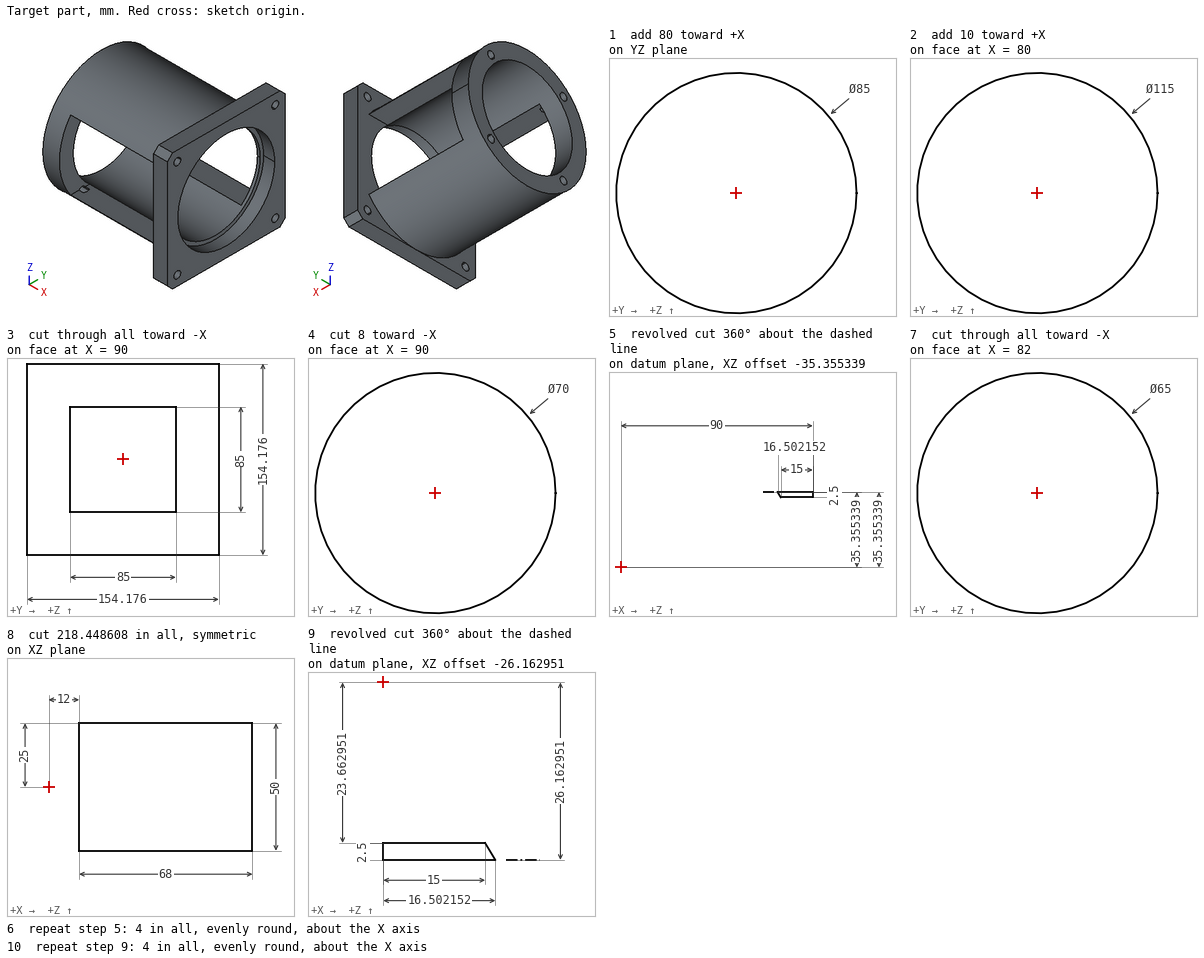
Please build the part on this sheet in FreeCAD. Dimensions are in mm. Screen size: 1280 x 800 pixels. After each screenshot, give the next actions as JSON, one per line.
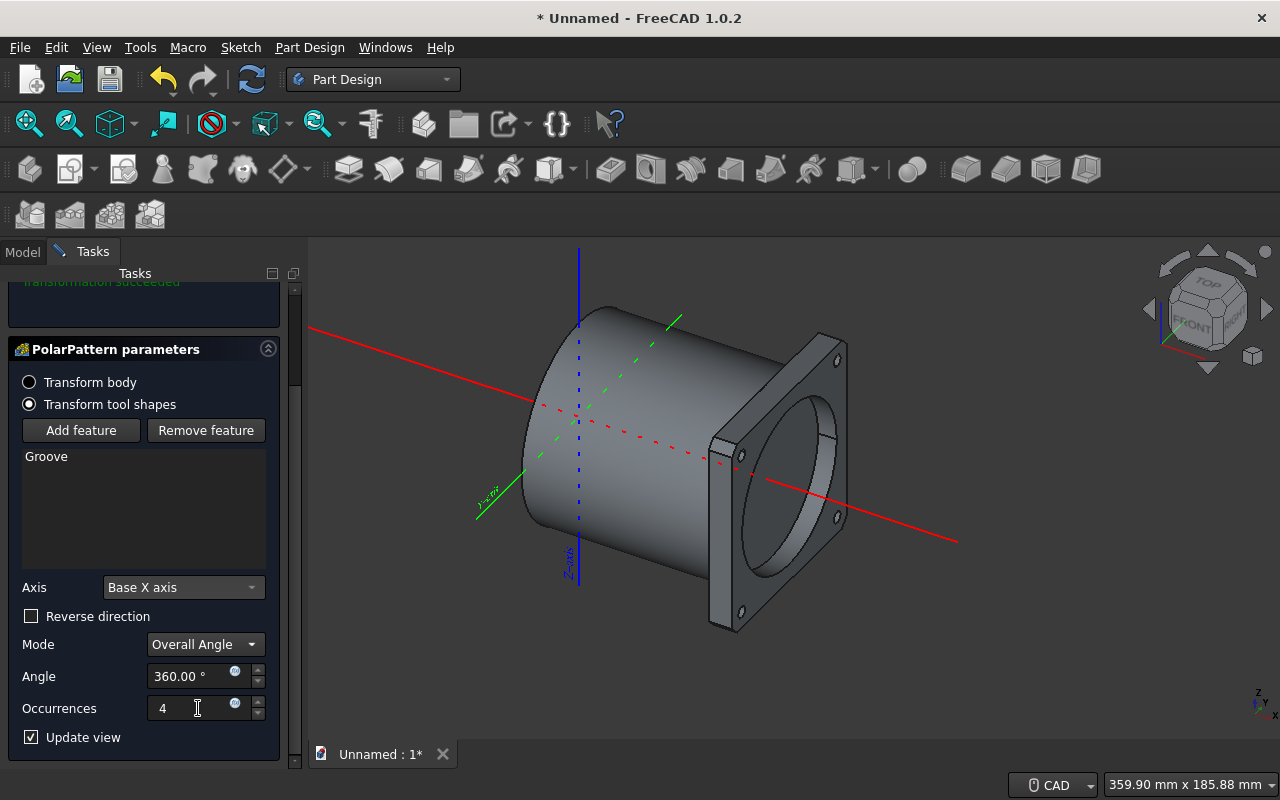
{"action": "scroll", "coordinate": [295, 526], "scroll_direction": "up", "scroll_amount": 3}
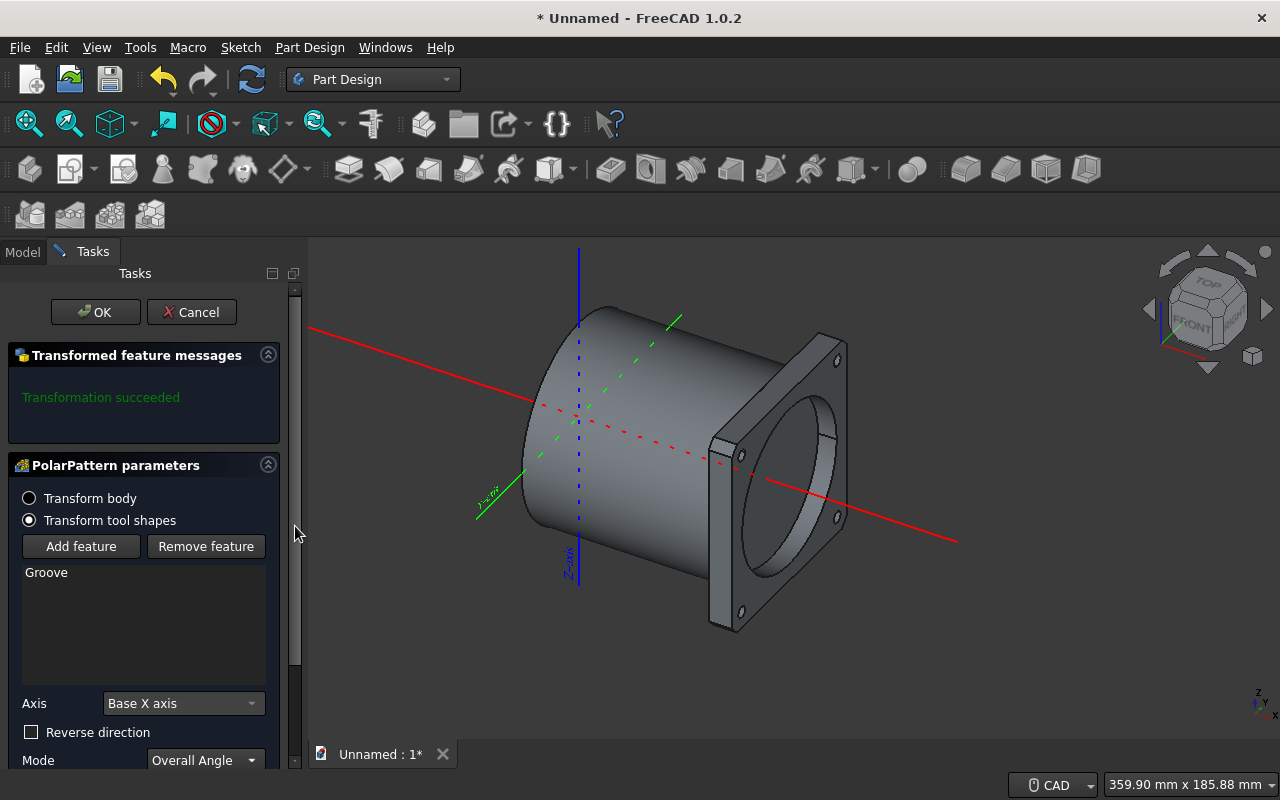
{"action": "left_click", "coordinate": [96, 312]}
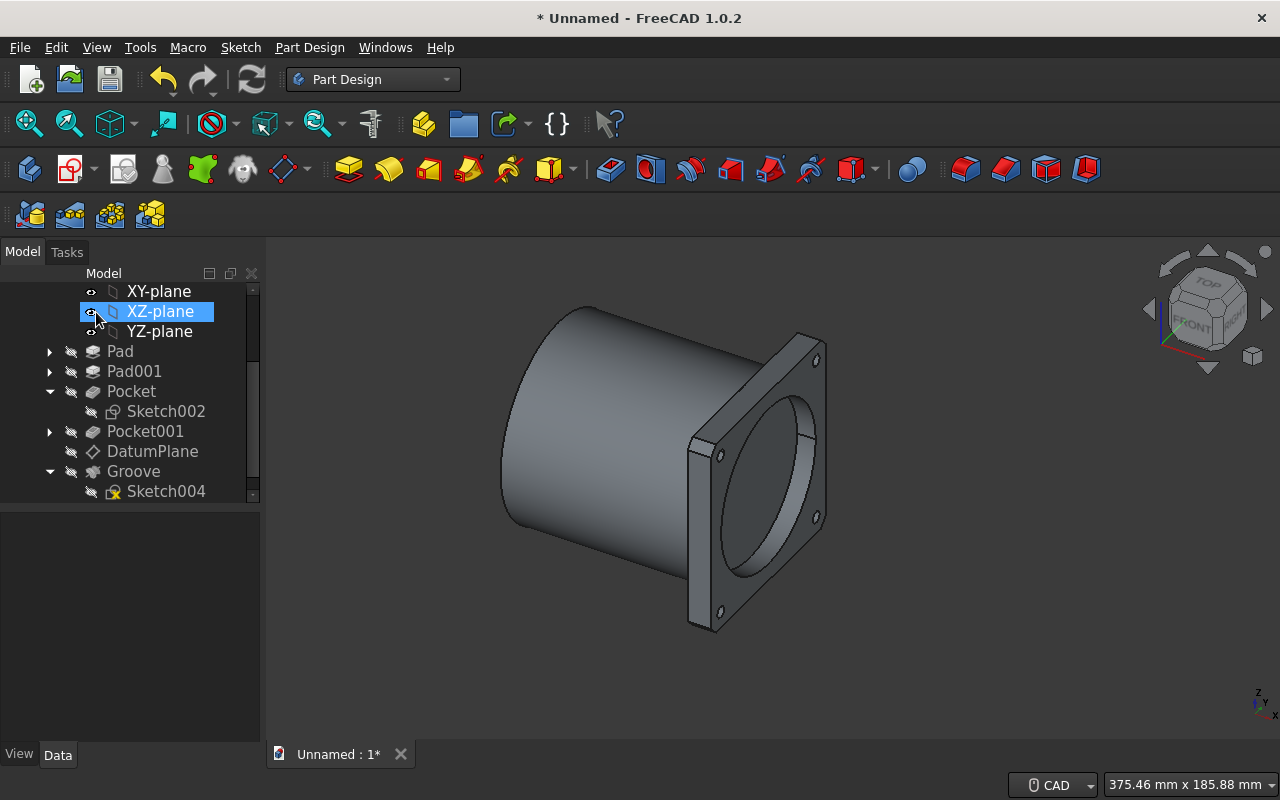
{"action": "left_click", "coordinate": [750, 479]}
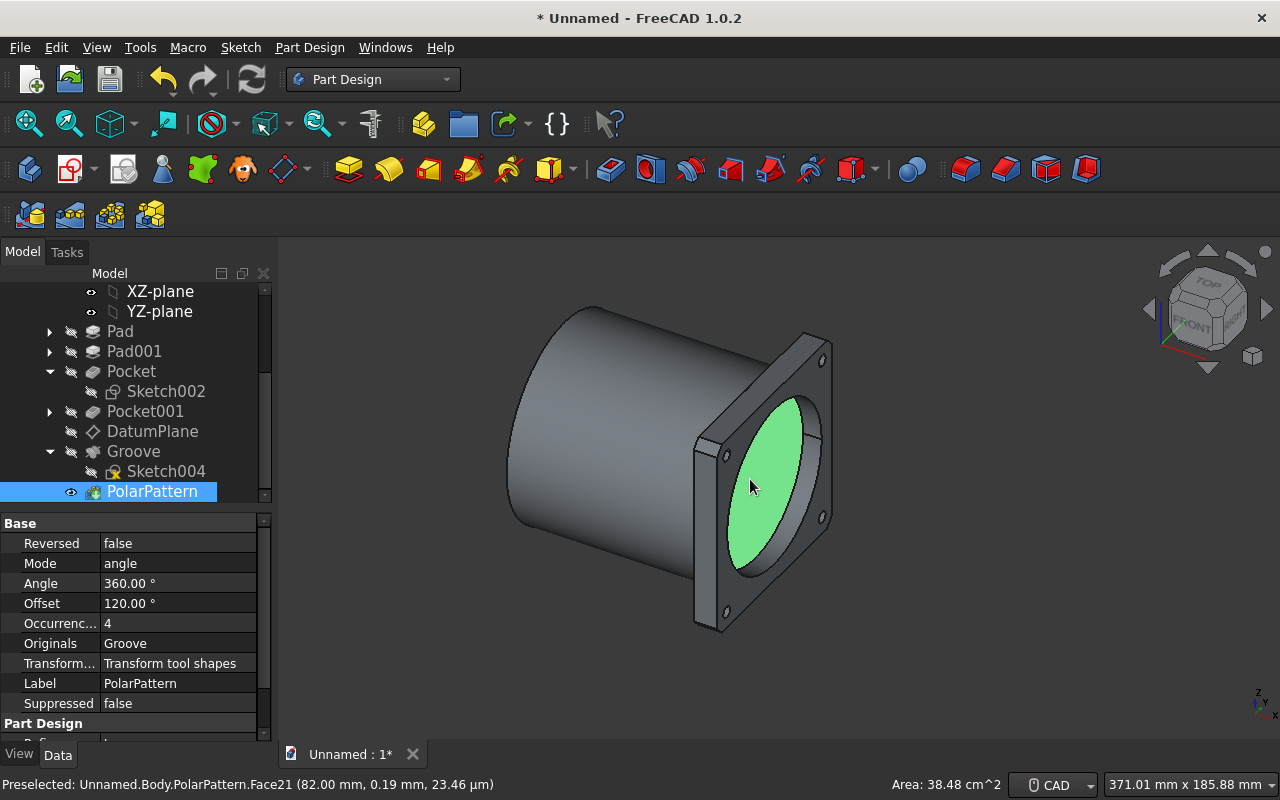
{"action": "left_click", "coordinate": [70, 170]}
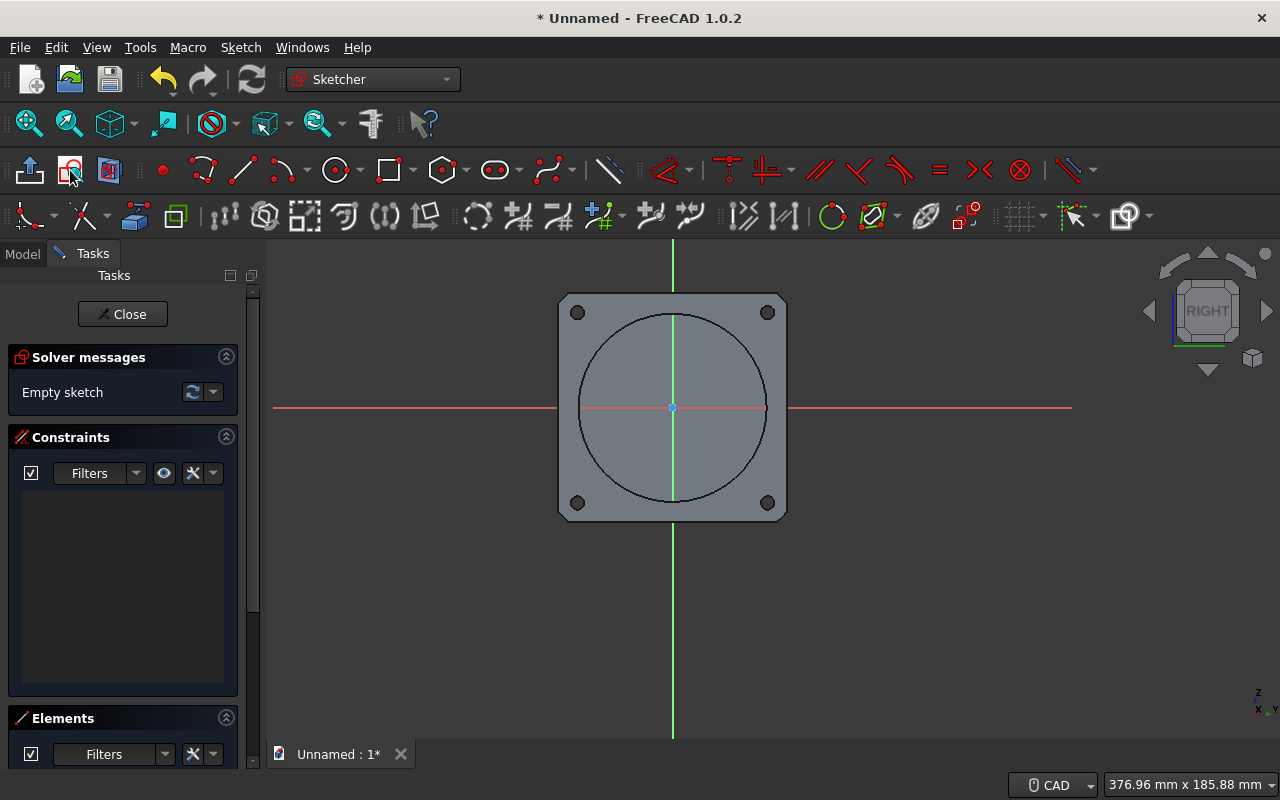
{"action": "scroll", "coordinate": [634, 309], "scroll_direction": "up", "scroll_amount": 3}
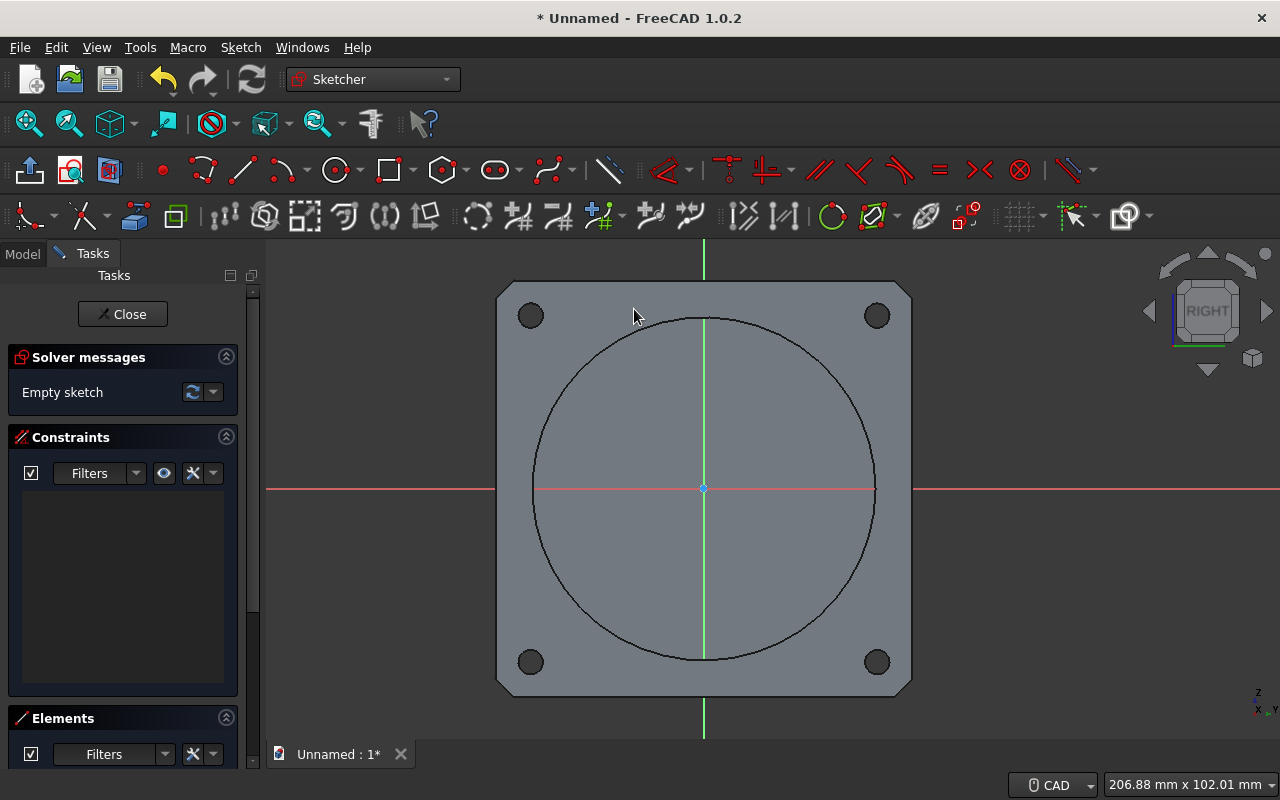
{"action": "left_click", "coordinate": [336, 170]}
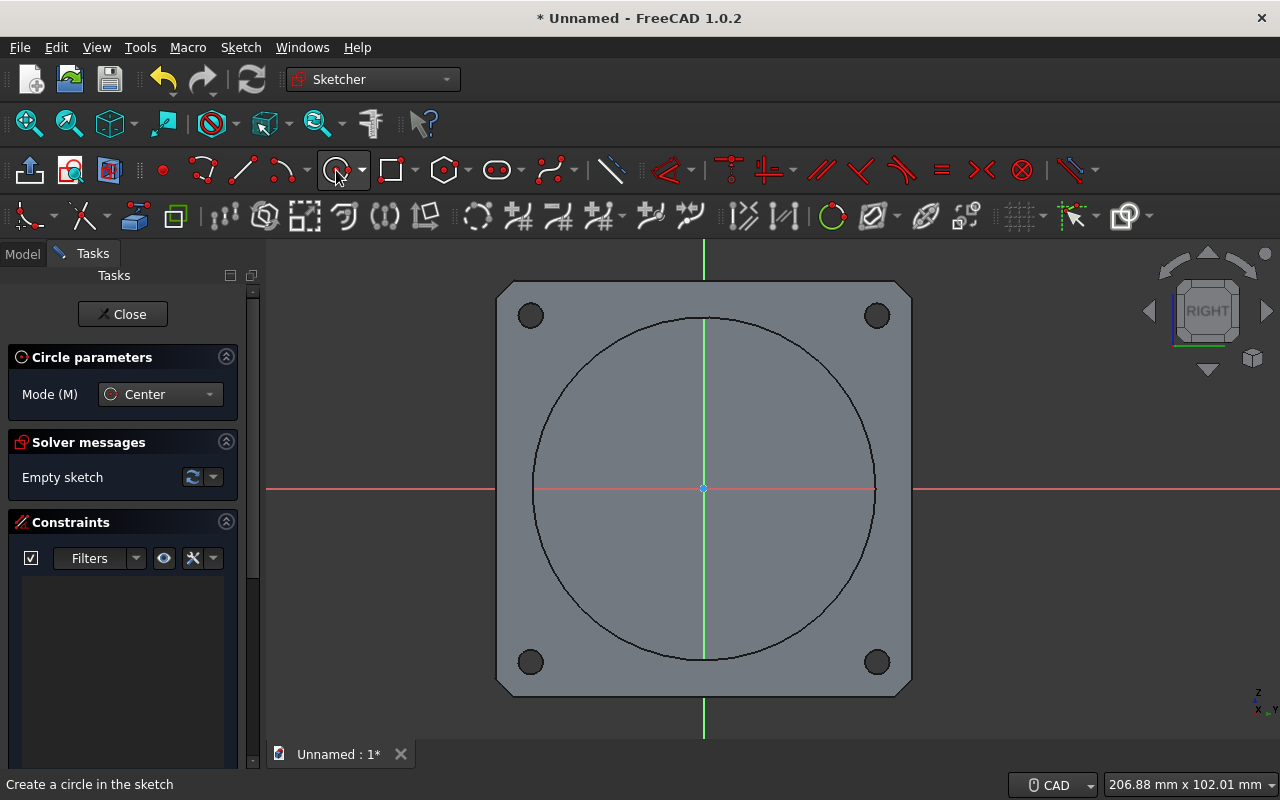
{"action": "left_click", "coordinate": [704, 489]}
{"action": "mouse_move", "coordinate": [817, 376]}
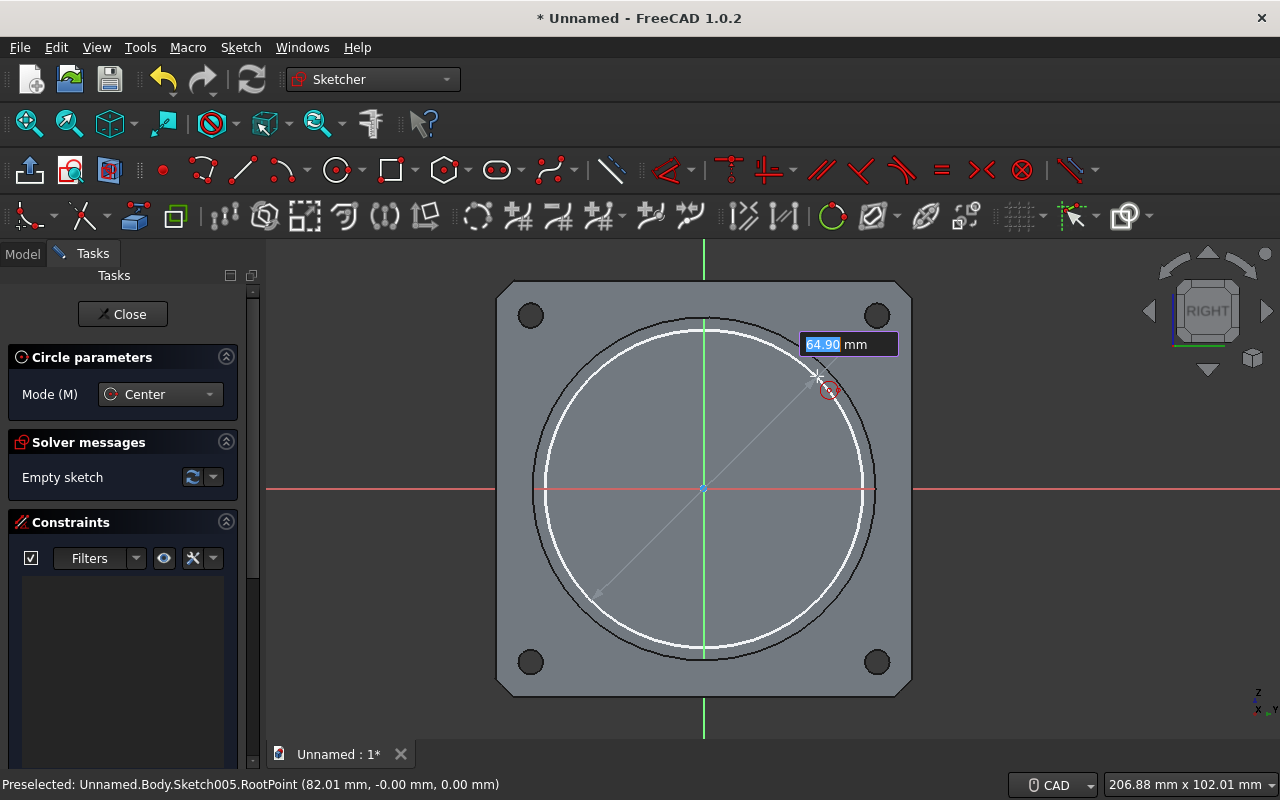
{"action": "type", "text": "65"}
{"action": "key", "text": "Return"}
{"action": "key", "text": "Escape"}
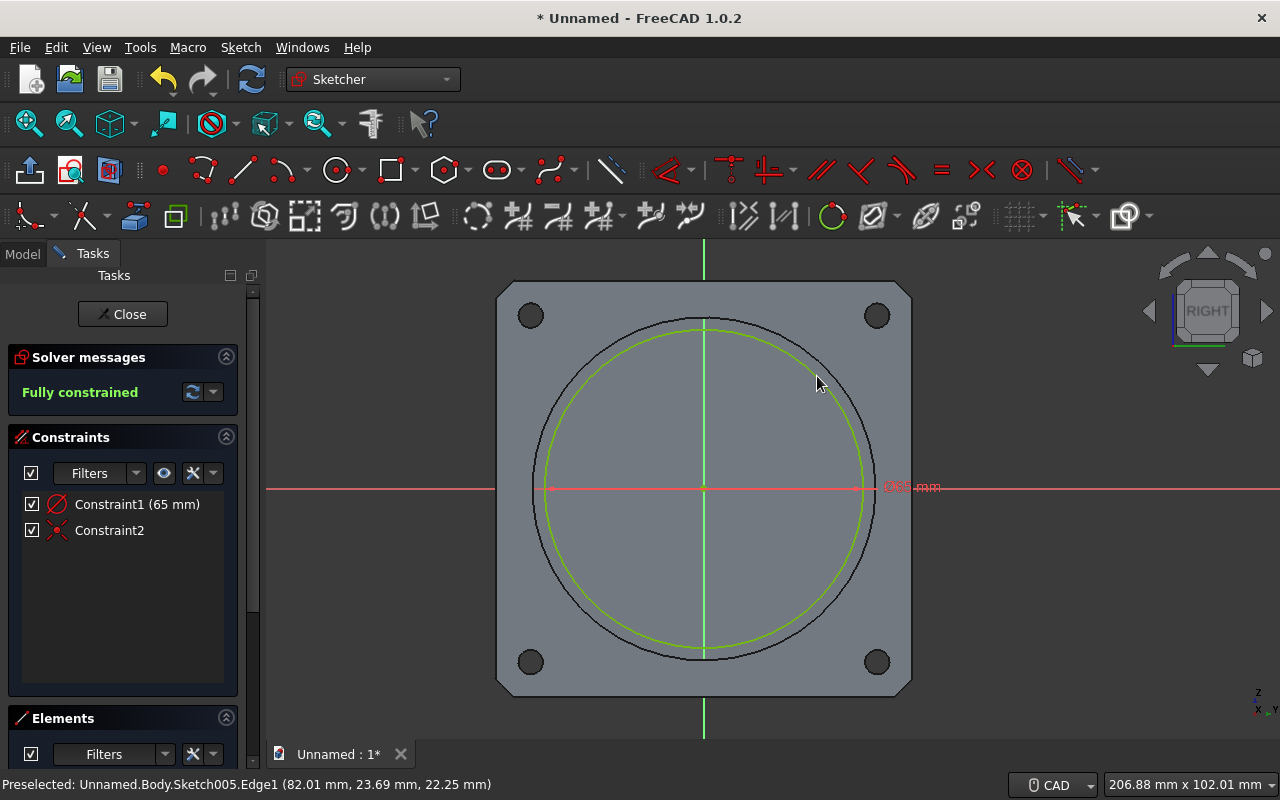
{"action": "left_click", "coordinate": [123, 314]}